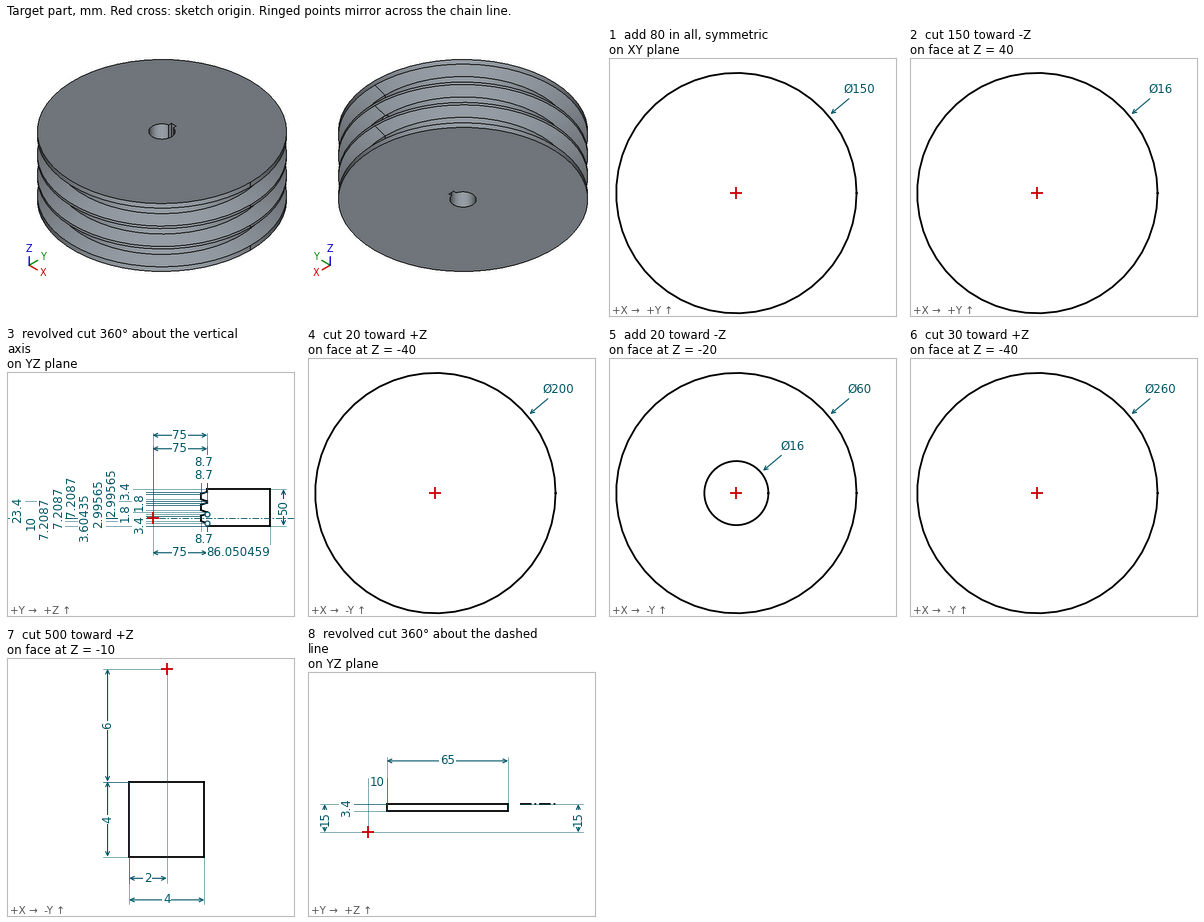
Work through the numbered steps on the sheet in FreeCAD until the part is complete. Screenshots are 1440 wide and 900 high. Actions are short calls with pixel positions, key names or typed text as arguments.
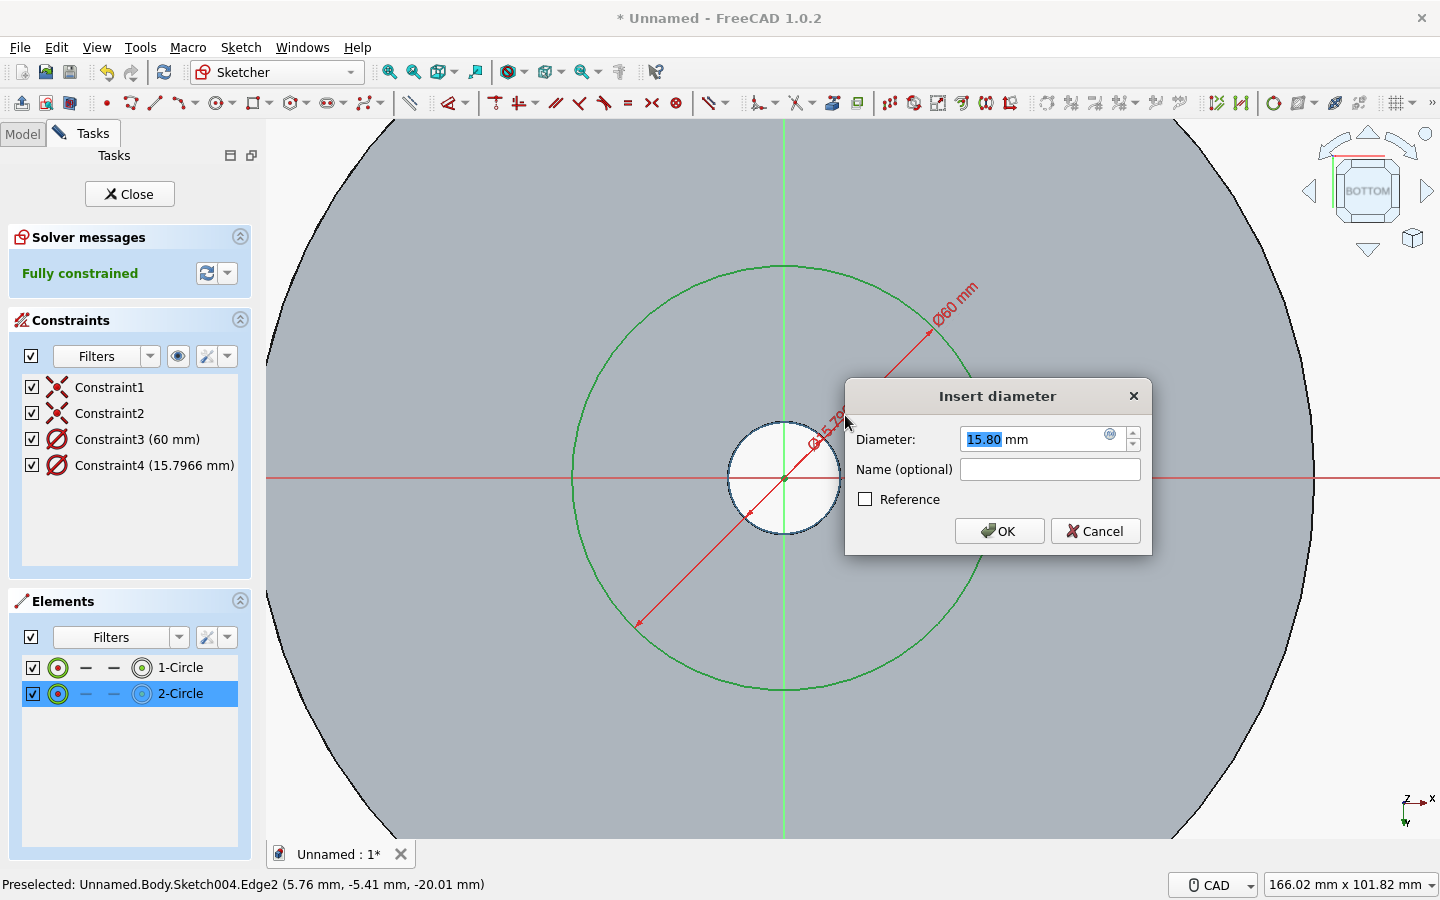
text(16)
key(Return)
key(Escape)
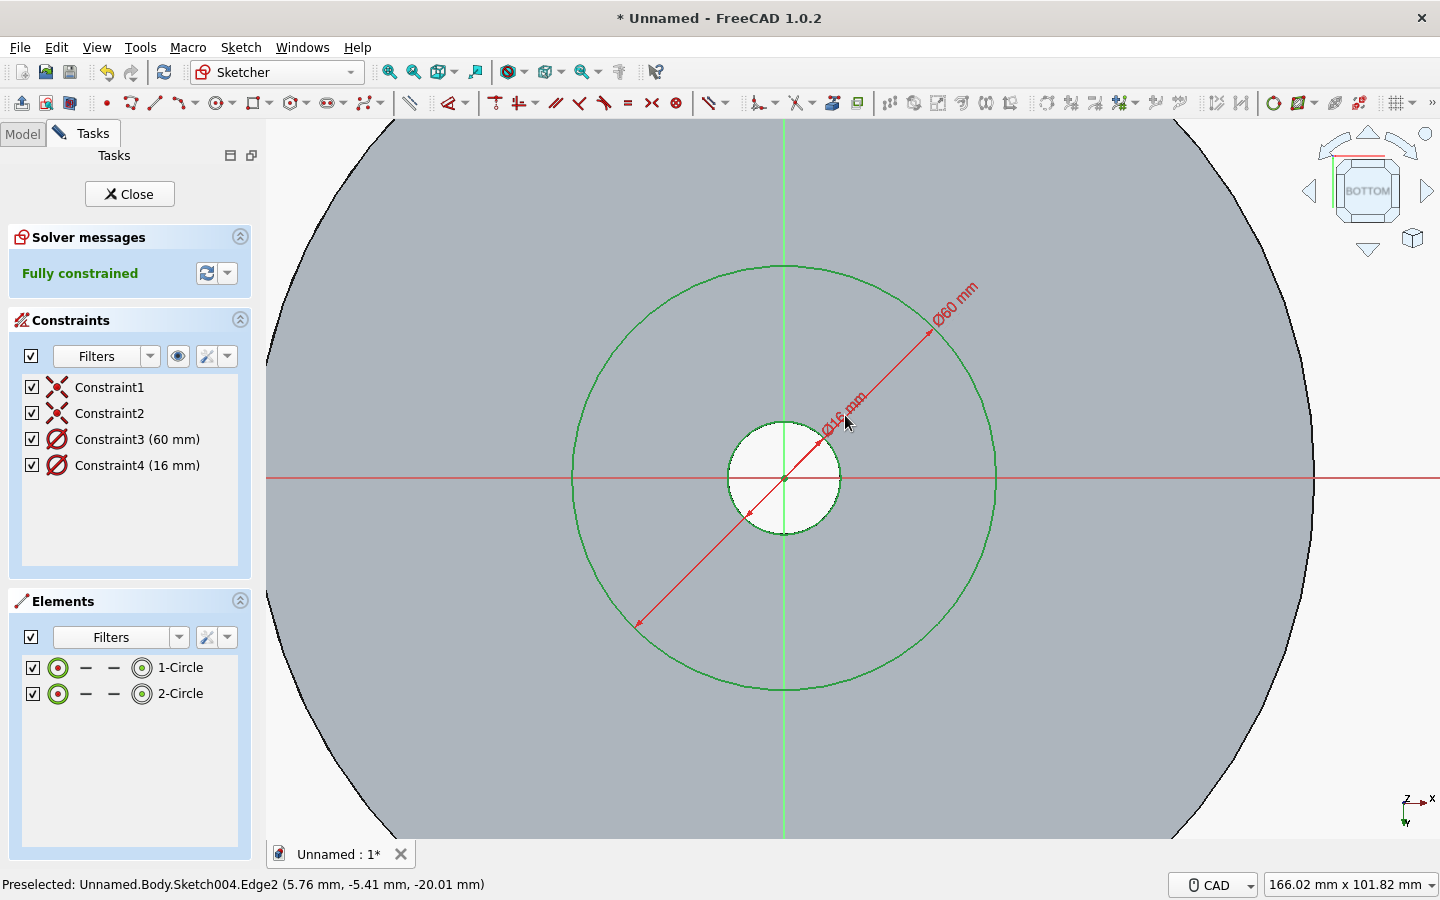
click(130, 194)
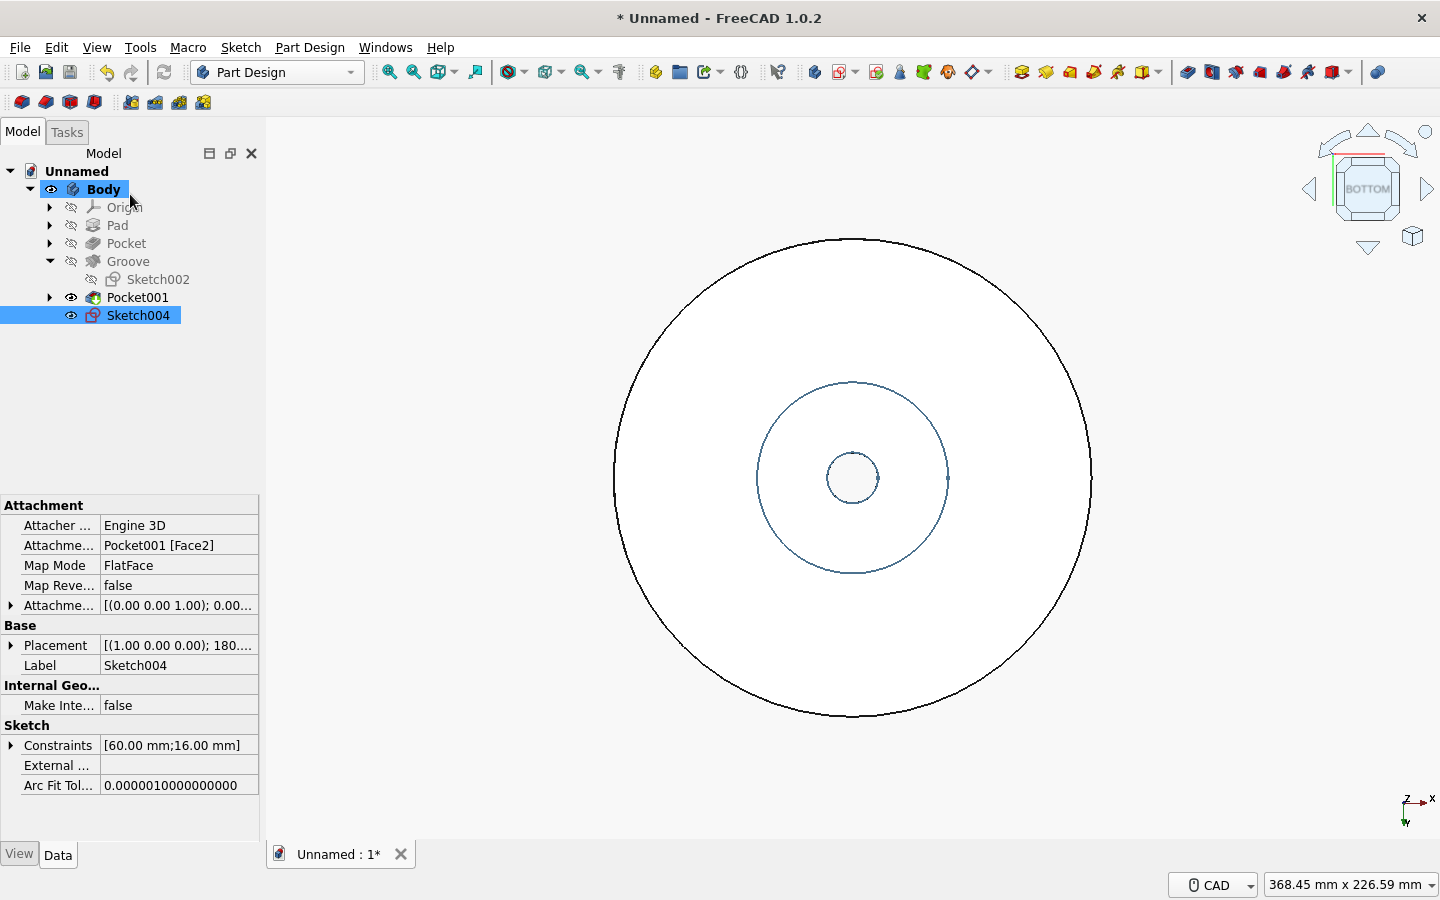
click(1022, 72)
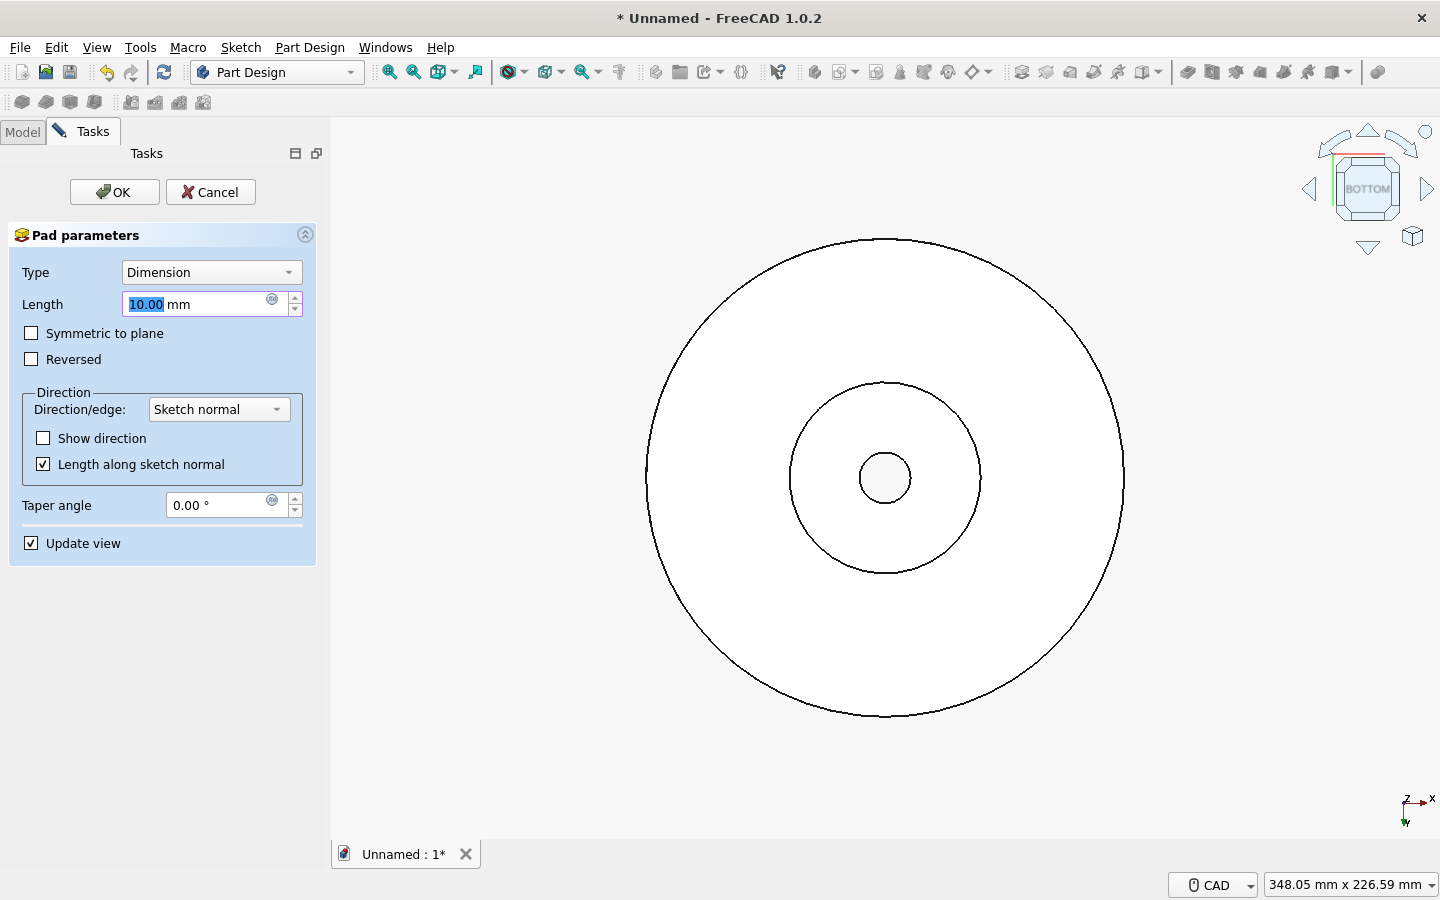
text(20)
key(Tab)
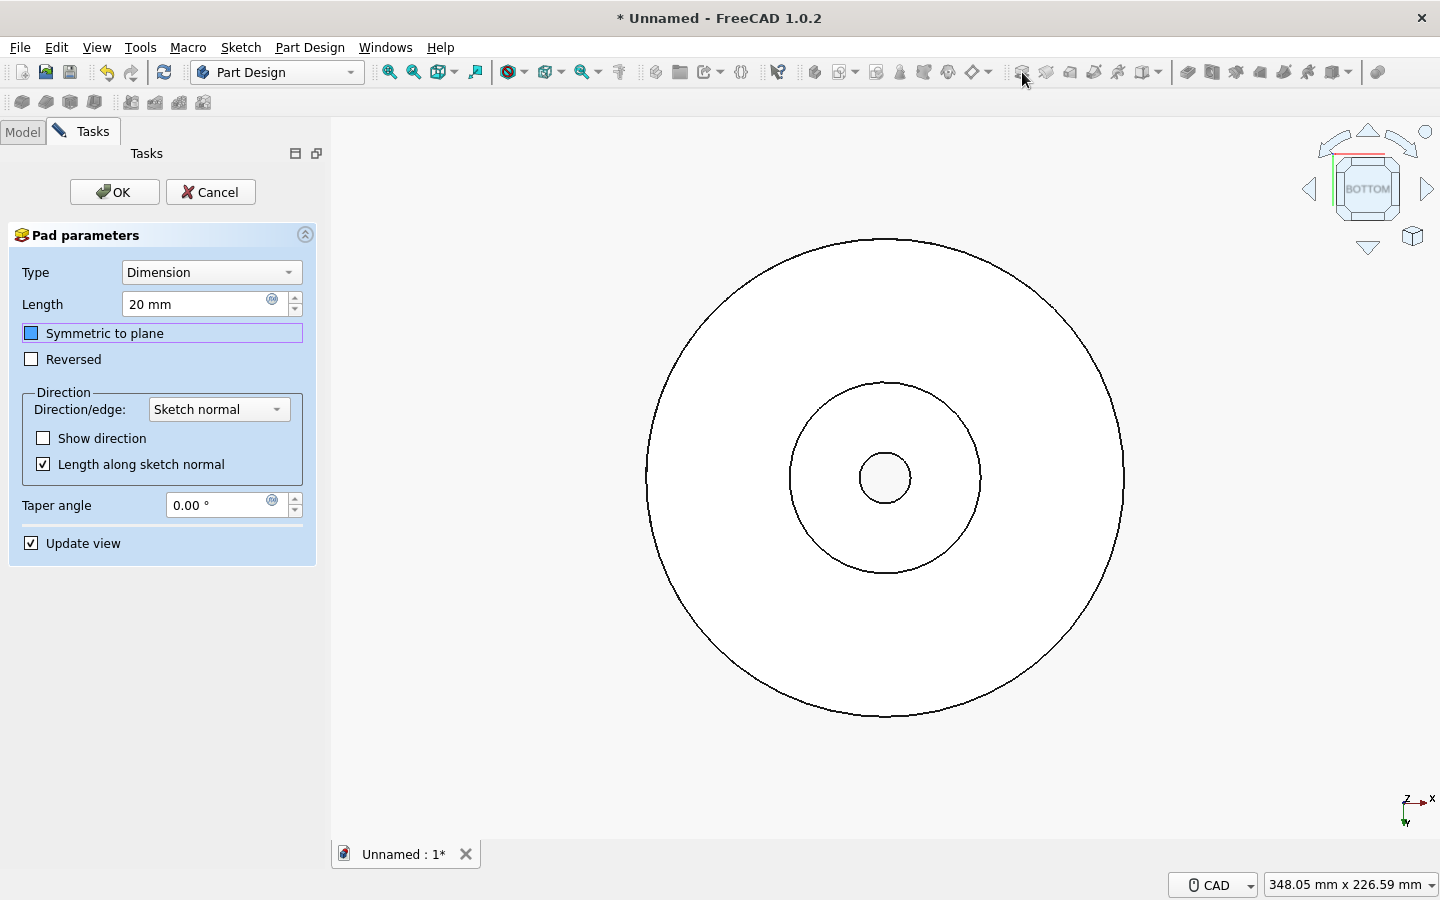
click(115, 192)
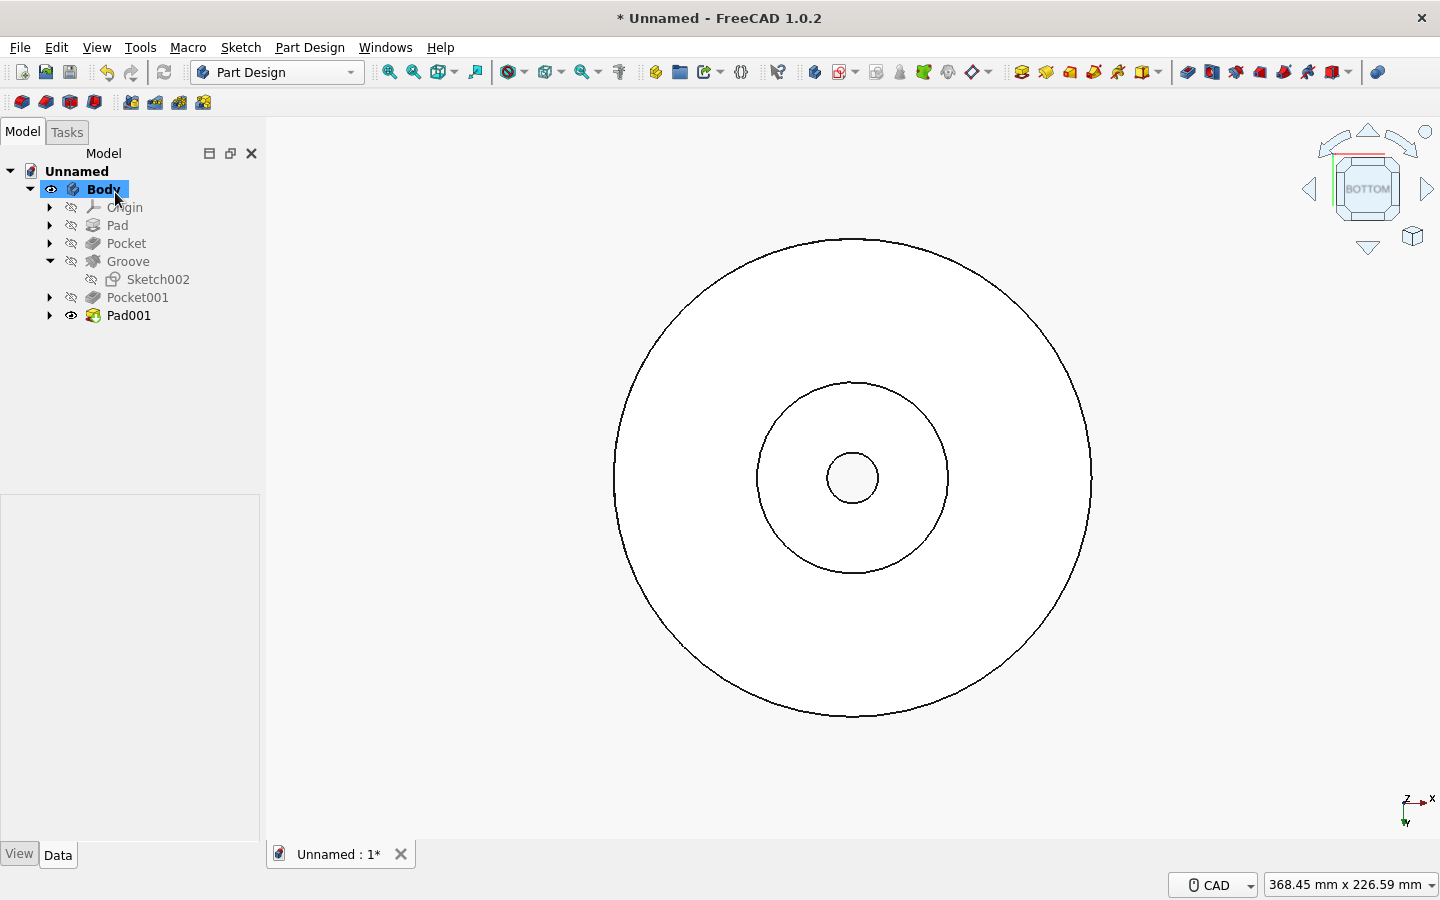
click(880, 422)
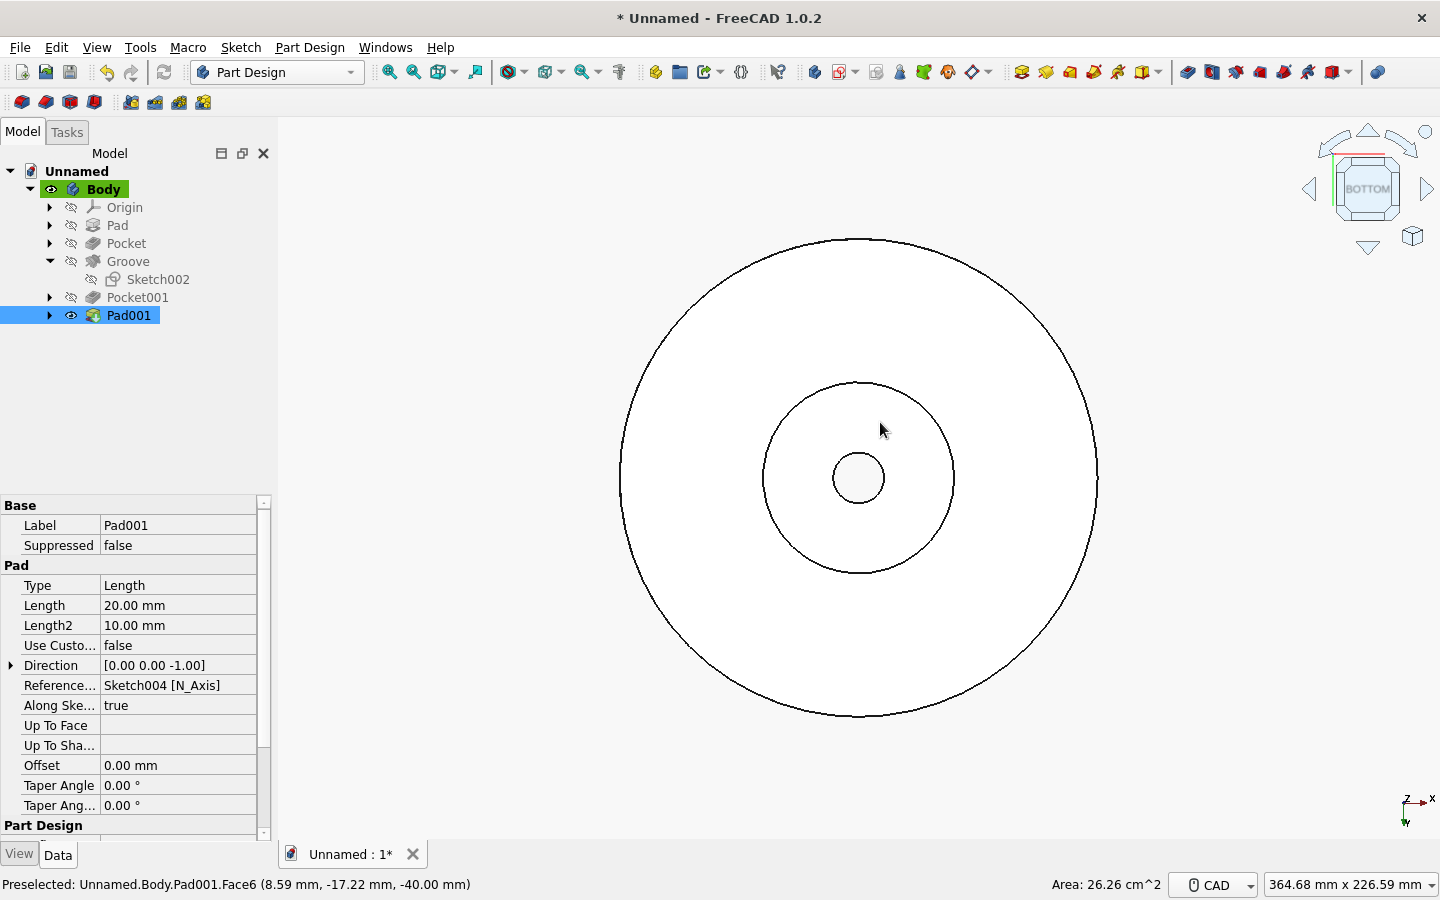
click(840, 72)